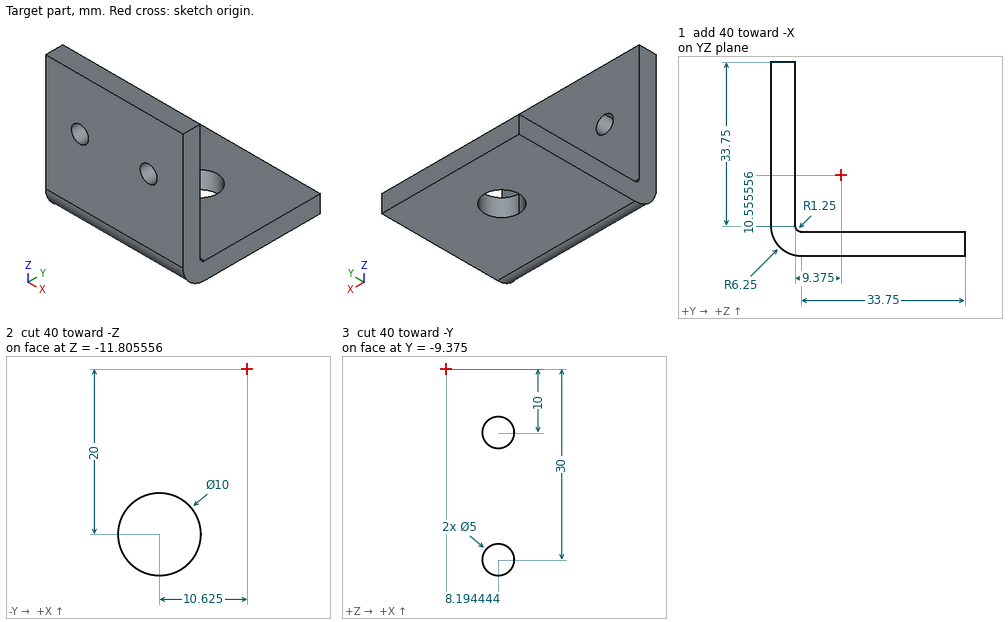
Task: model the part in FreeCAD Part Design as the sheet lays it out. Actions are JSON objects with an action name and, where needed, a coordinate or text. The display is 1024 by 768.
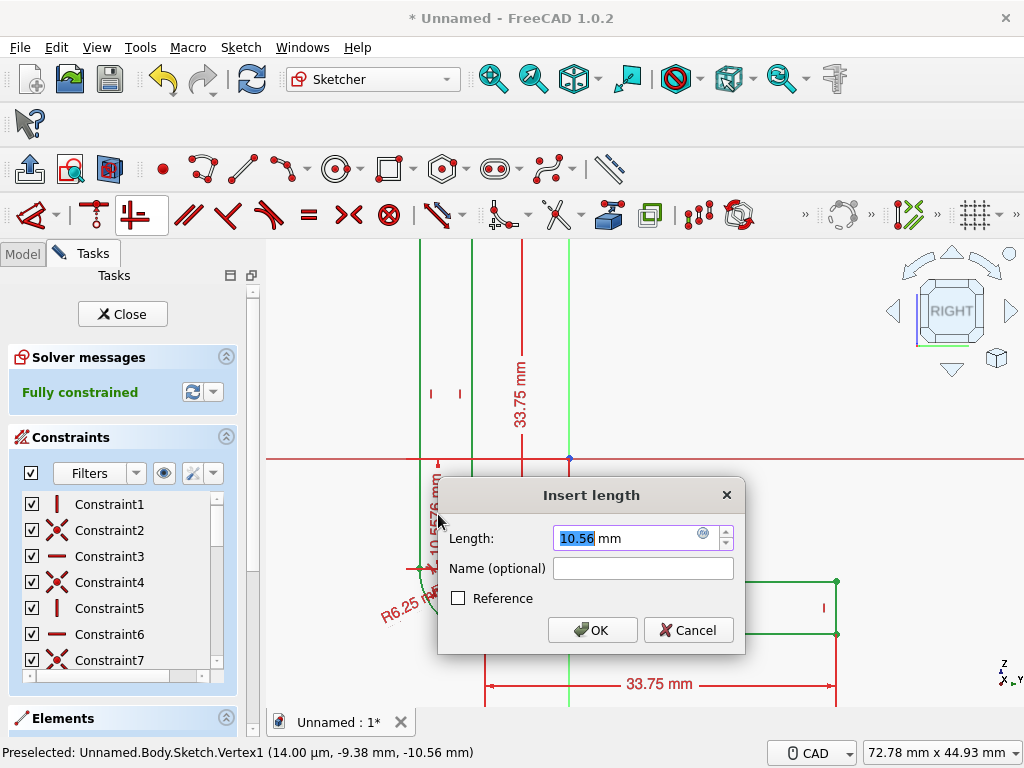
{"action": "type", "text": "10.555556"}
{"action": "key", "text": "Return"}
{"action": "key", "text": "Escape"}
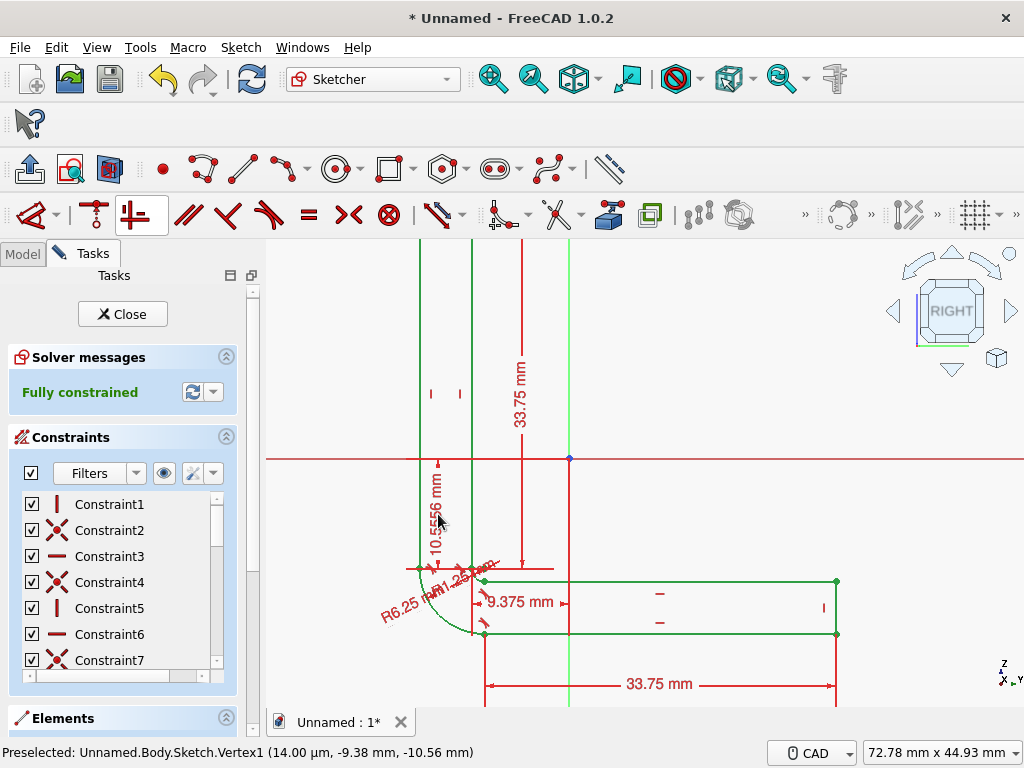
{"action": "left_click", "coordinate": [123, 314]}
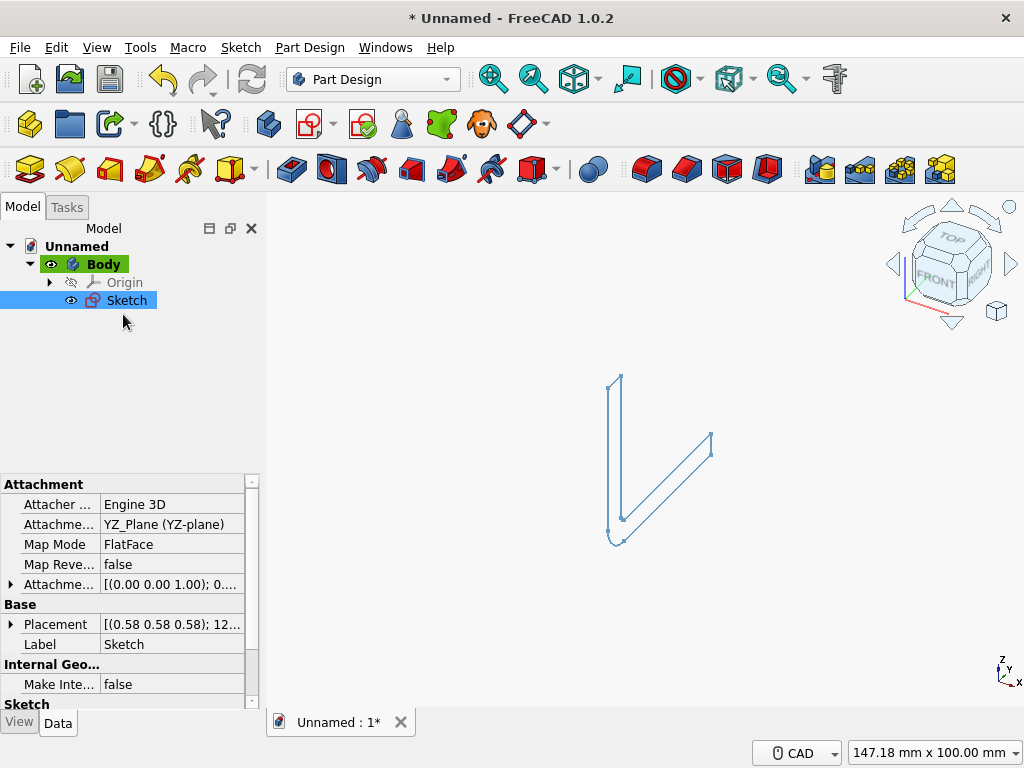
{"action": "left_click", "coordinate": [30, 170]}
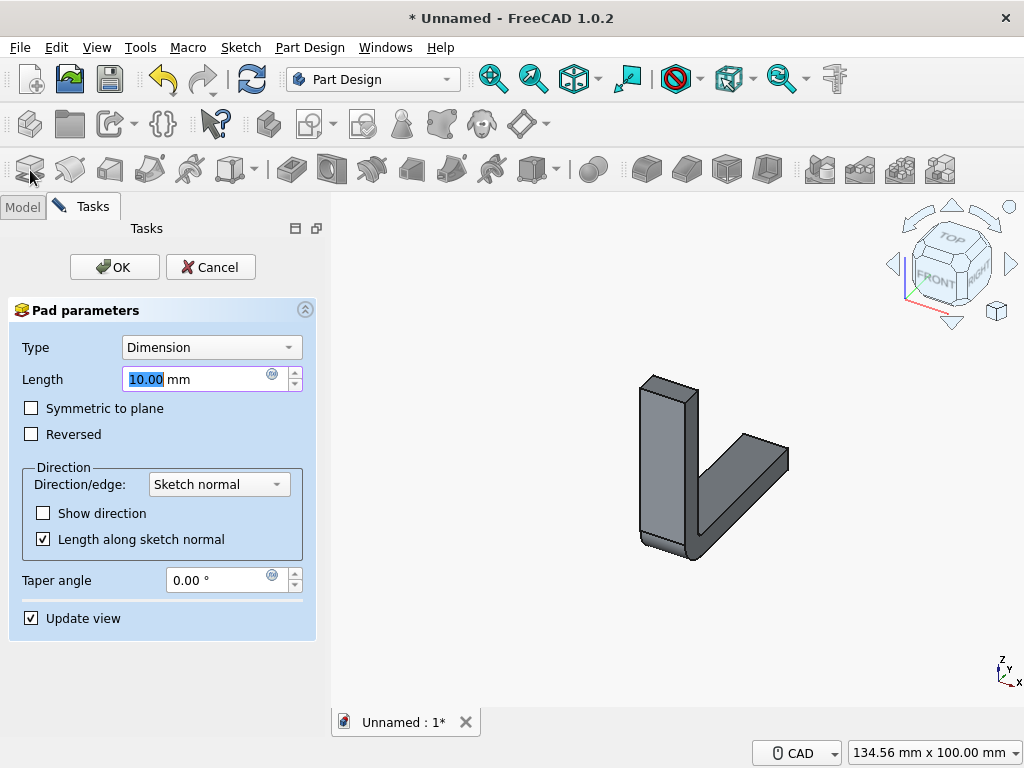
{"action": "type", "text": "40"}
{"action": "key", "text": "Tab"}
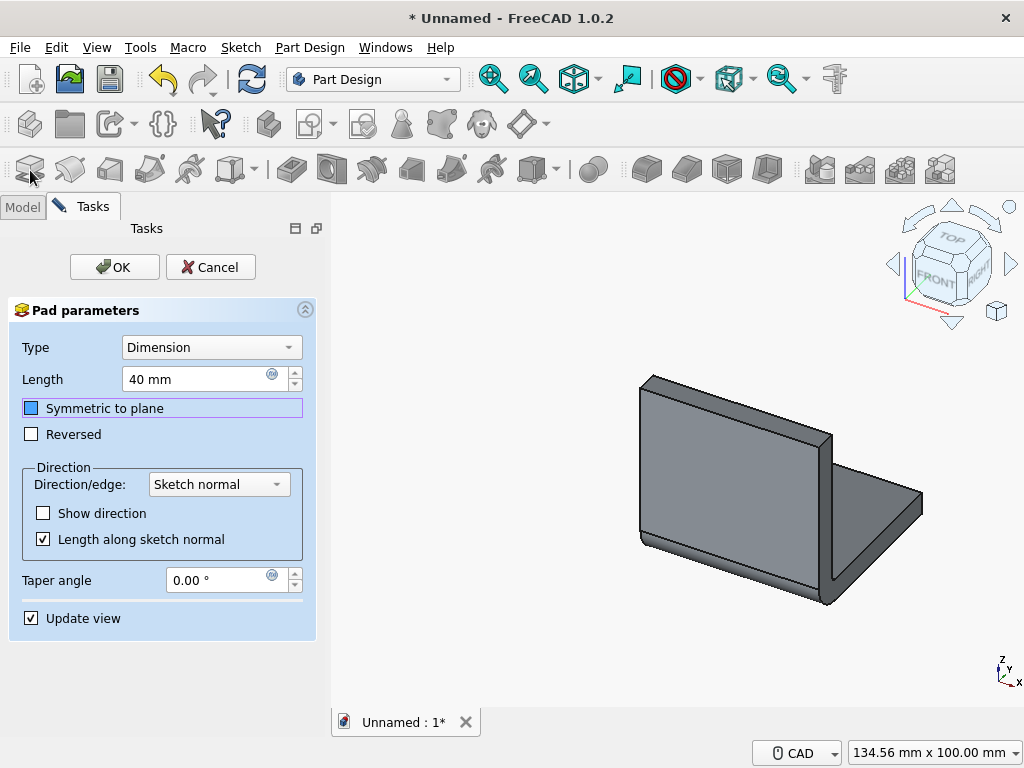
{"action": "left_click", "coordinate": [30, 434]}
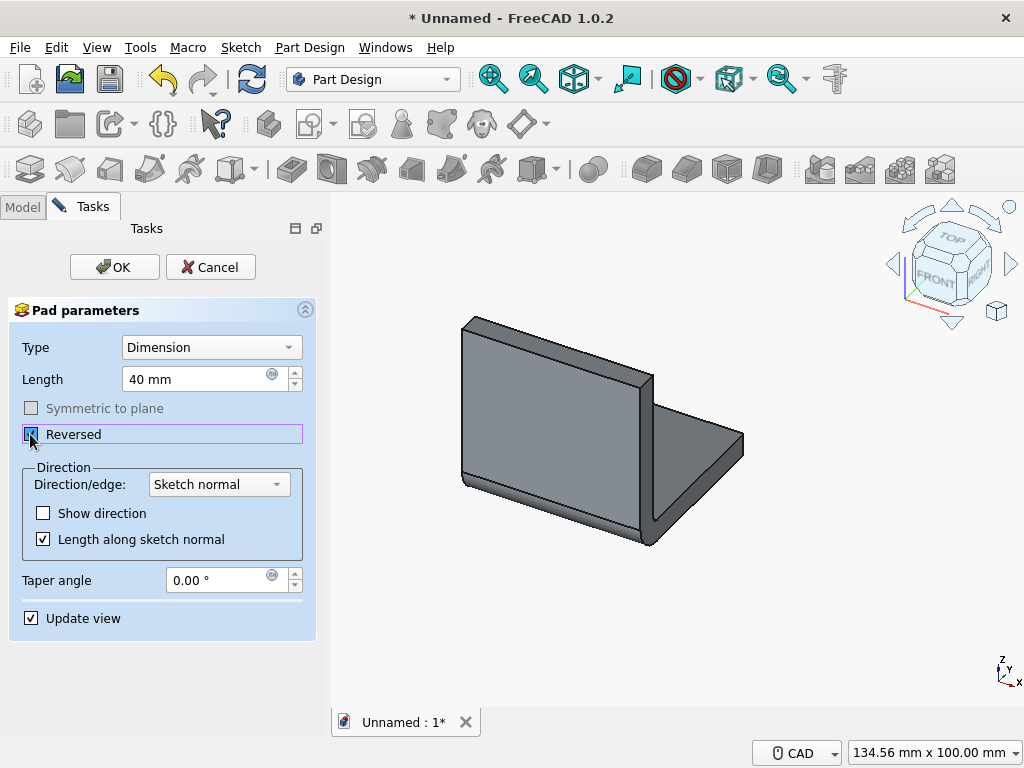
{"action": "left_click", "coordinate": [115, 267]}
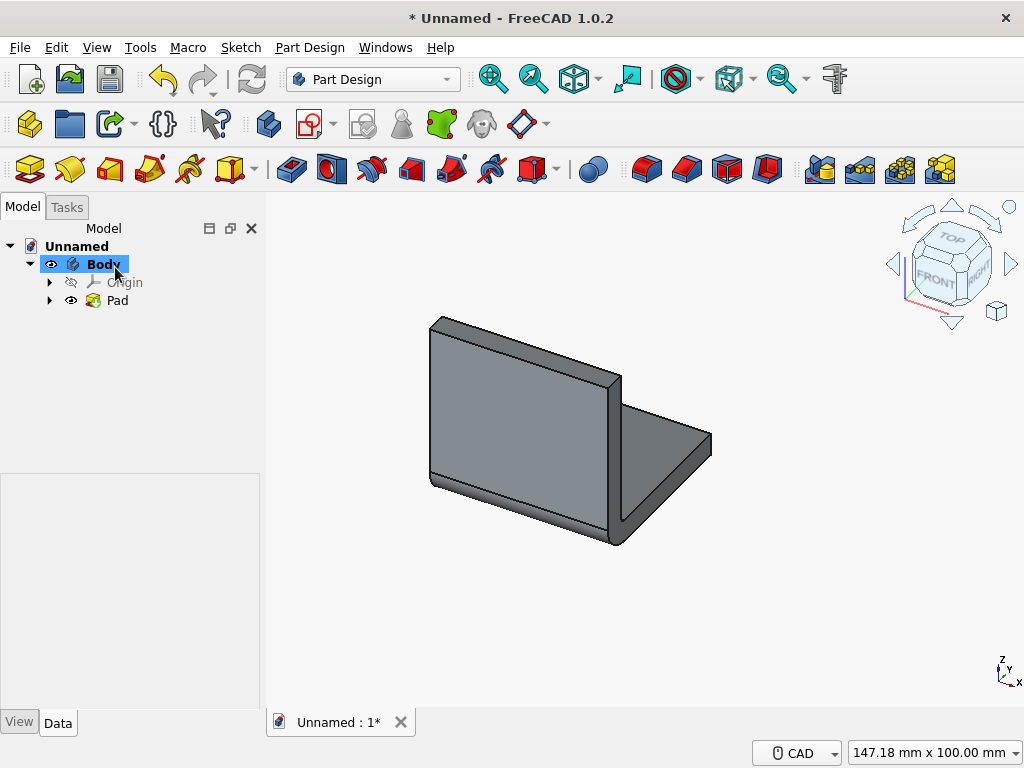
{"action": "key", "text": "0"}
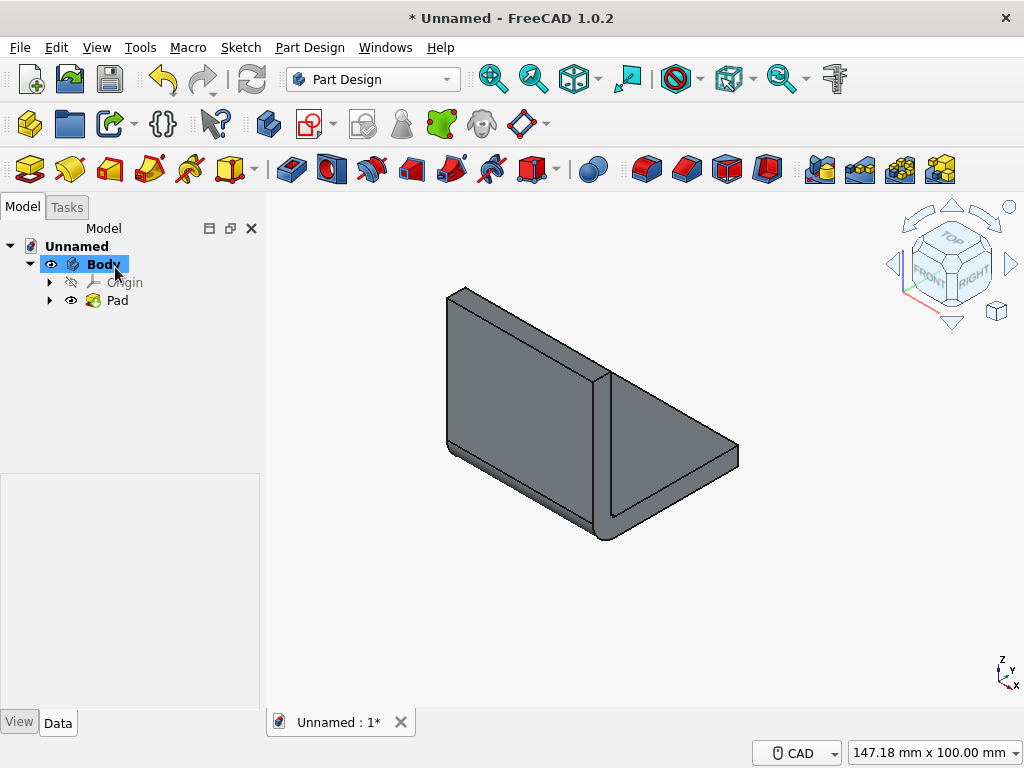
{"action": "left_click", "coordinate": [625, 450]}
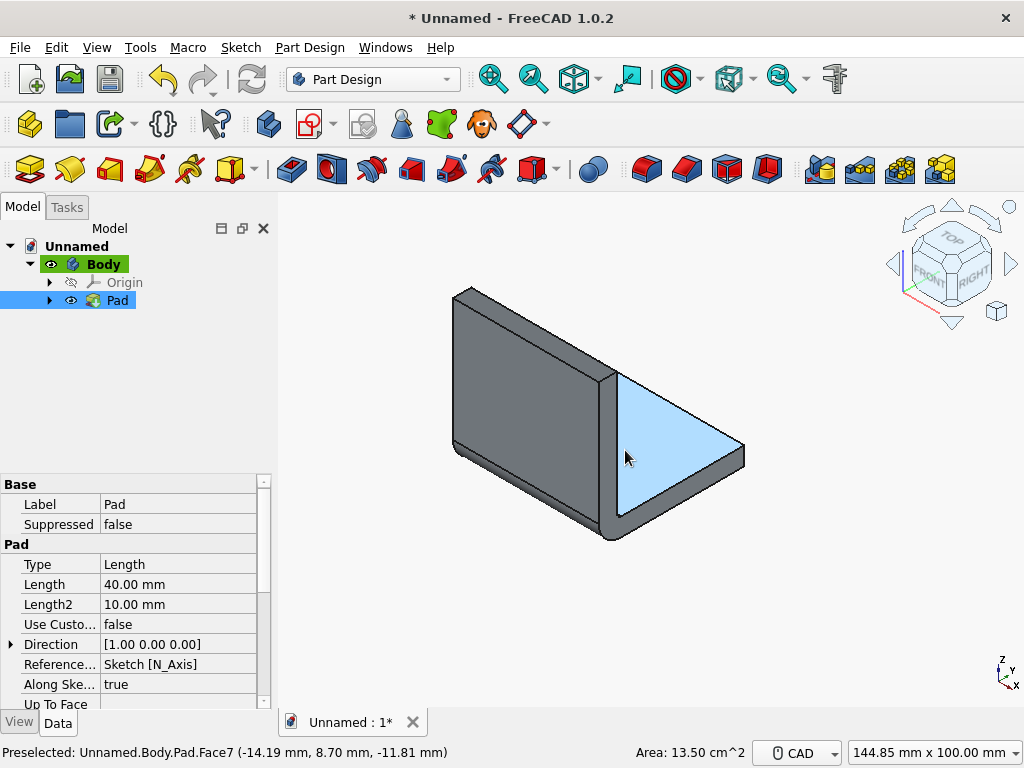
{"action": "left_click", "coordinate": [310, 124]}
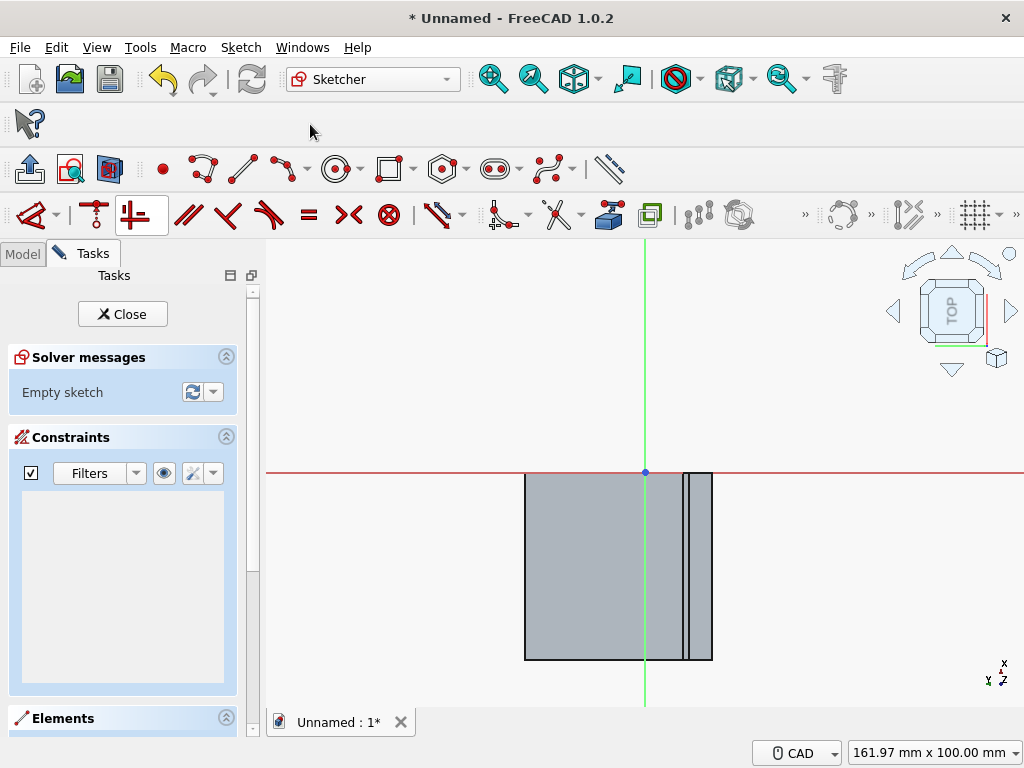
{"action": "scroll", "coordinate": [599, 585], "scroll_direction": "up", "scroll_amount": 9}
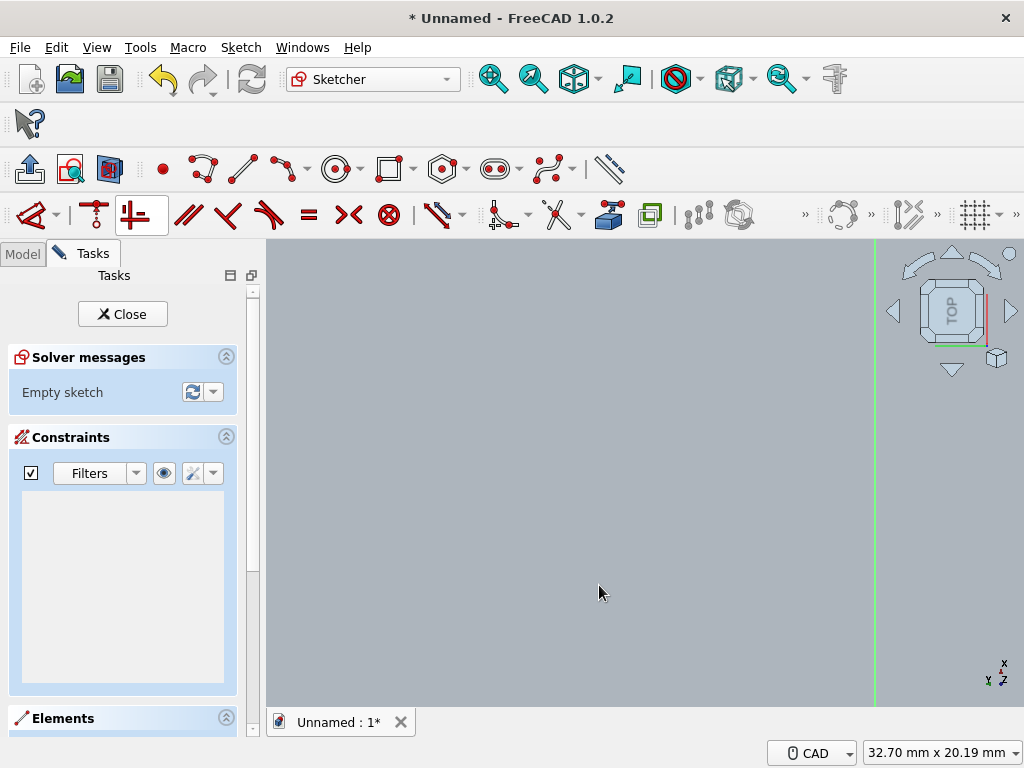
{"action": "key", "text": "g c"}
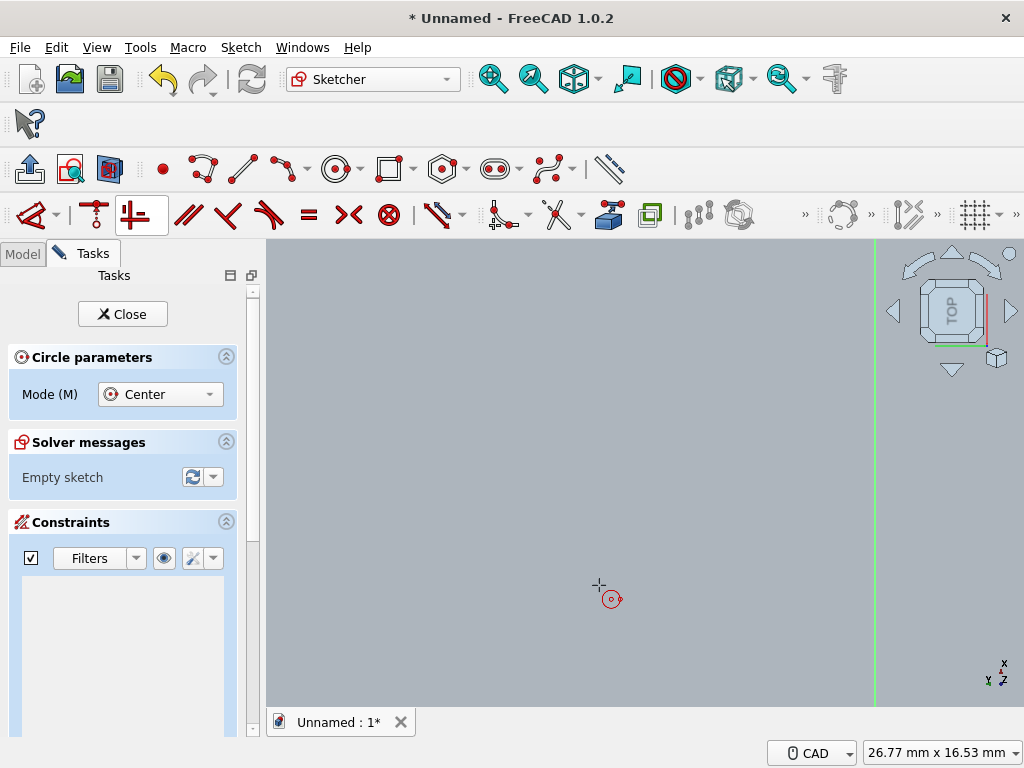
{"action": "left_click", "coordinate": [574, 470]}
{"action": "mouse_move", "coordinate": [674, 370]}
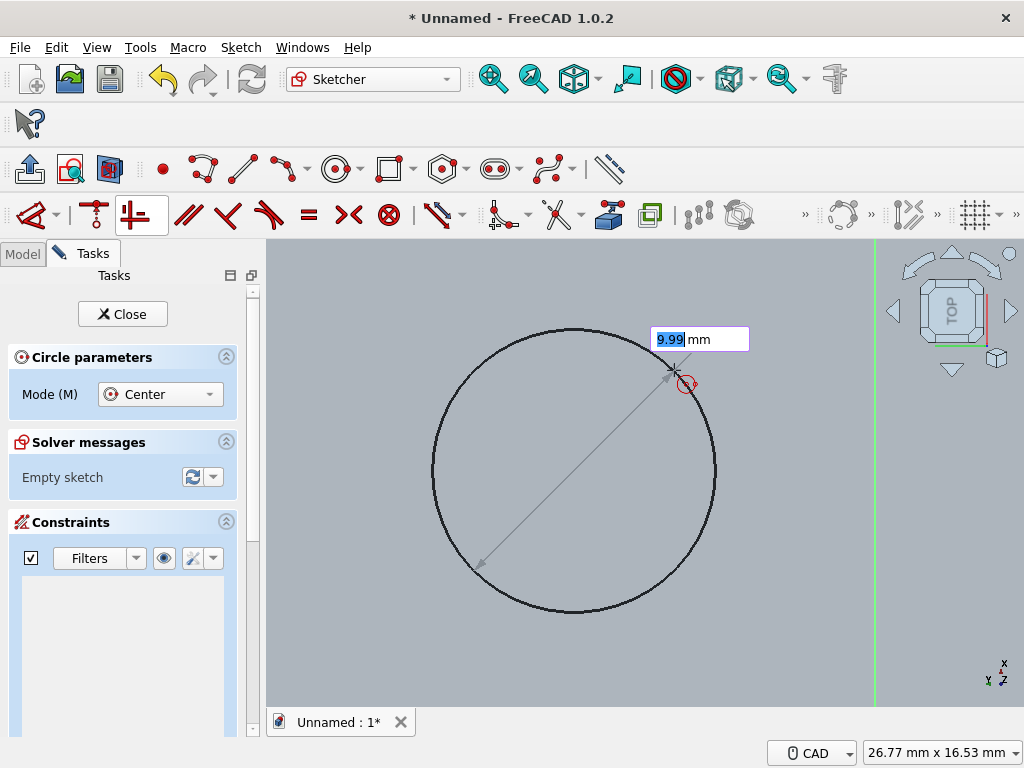
{"action": "type", "text": "10"}
{"action": "key", "text": "Return"}
{"action": "key", "text": "Escape"}